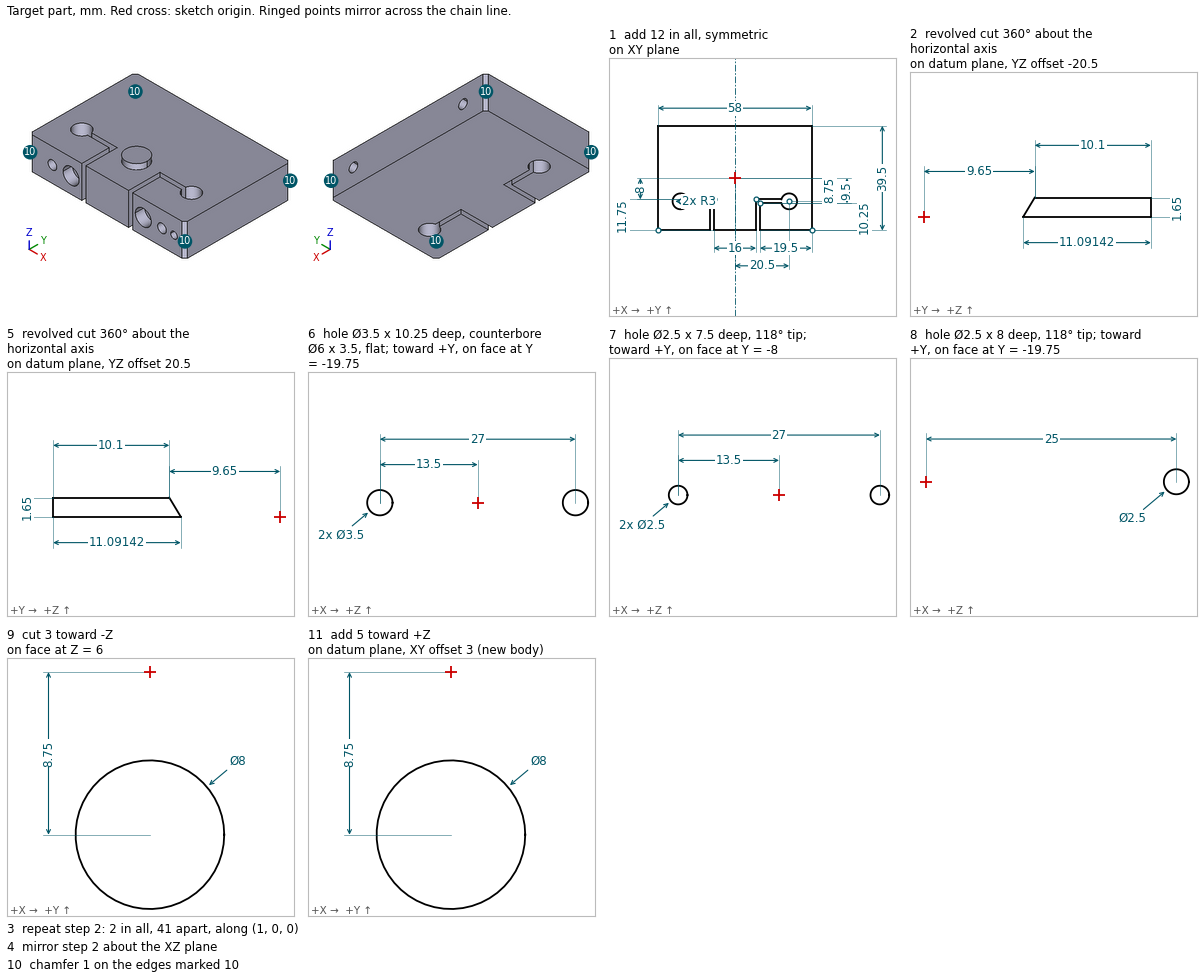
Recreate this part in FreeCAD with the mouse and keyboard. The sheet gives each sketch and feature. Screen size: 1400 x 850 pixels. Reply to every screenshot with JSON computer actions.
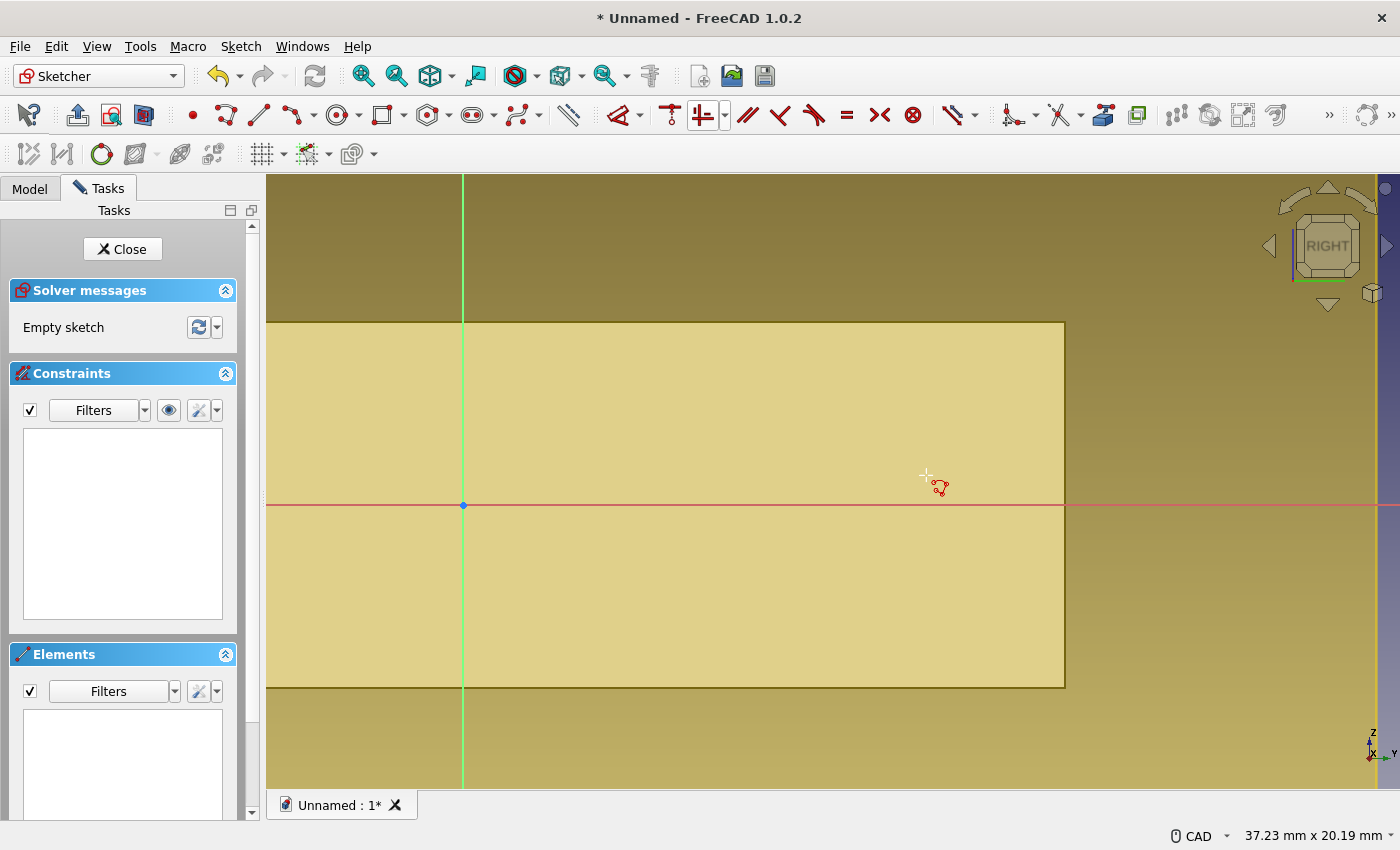
{"action": "left_click", "coordinate": [727, 505]}
{"action": "left_click", "coordinate": [1065, 496]}
{"action": "left_click", "coordinate": [1065, 455]}
{"action": "left_click", "coordinate": [757, 455]}
{"action": "left_click", "coordinate": [727, 505]}
{"action": "key", "text": "Escape"}
{"action": "key", "text": "Escape"}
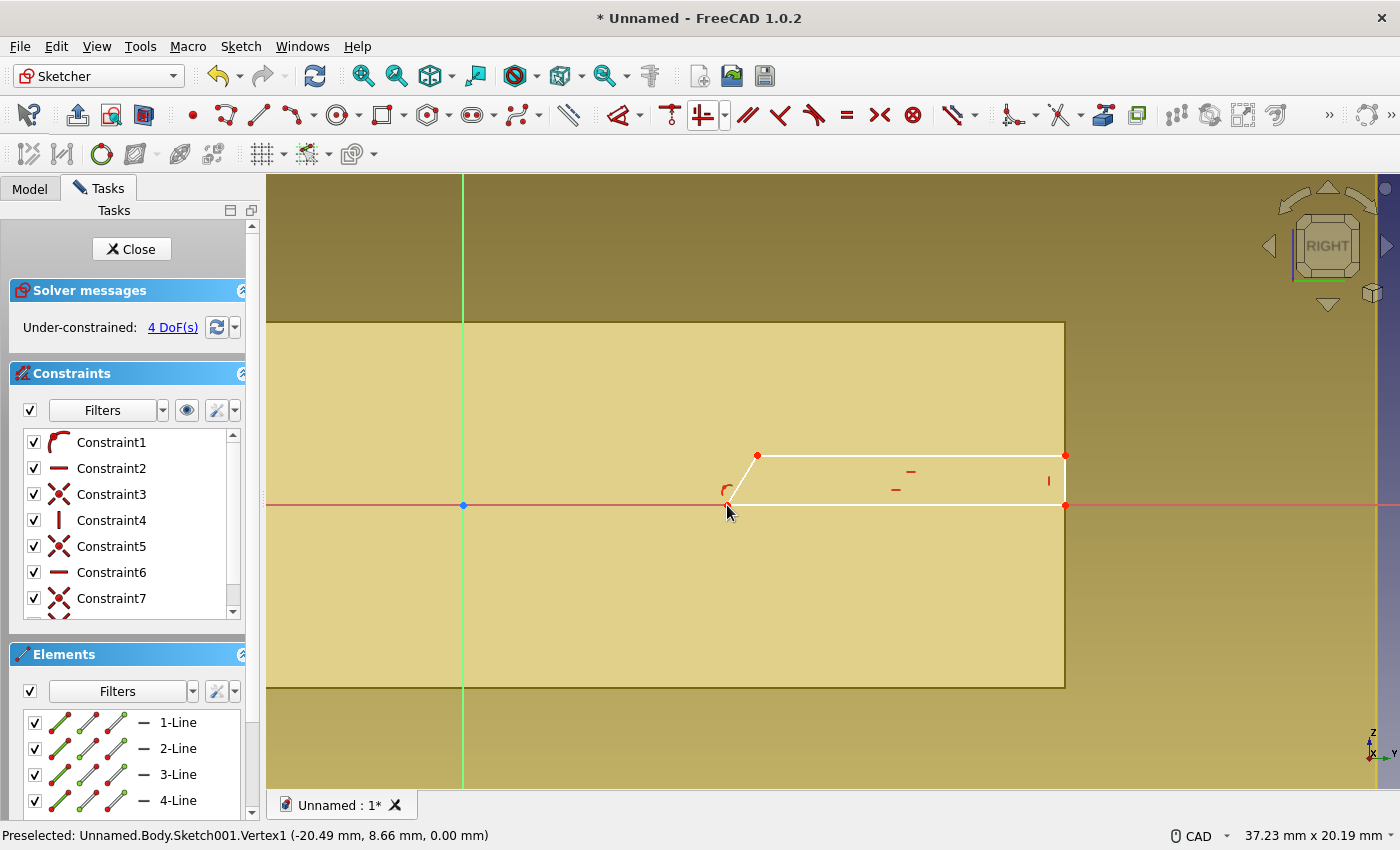
{"action": "left_click", "coordinate": [618, 116]}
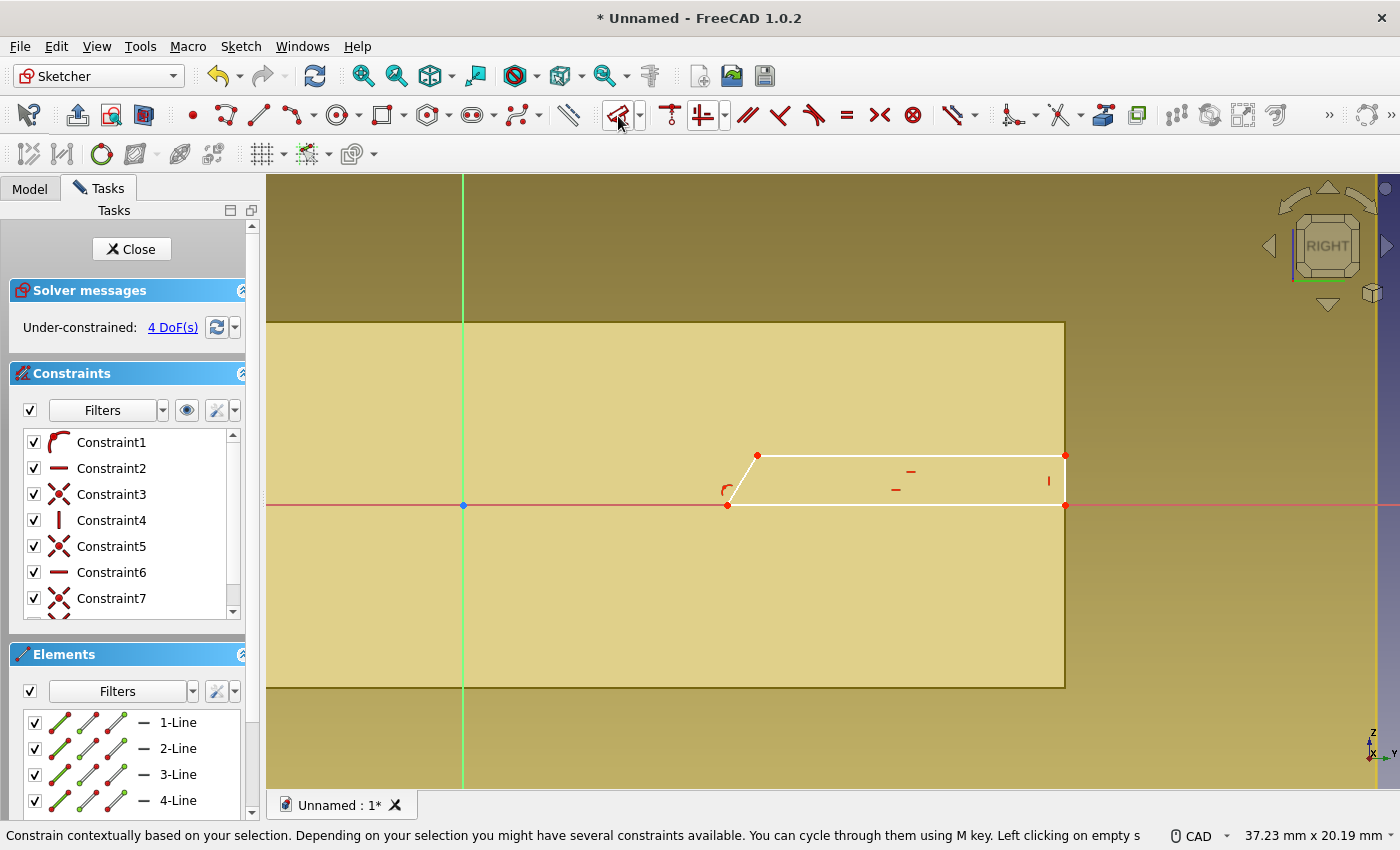
{"action": "left_click", "coordinate": [1065, 490]}
{"action": "left_click", "coordinate": [1099, 481]}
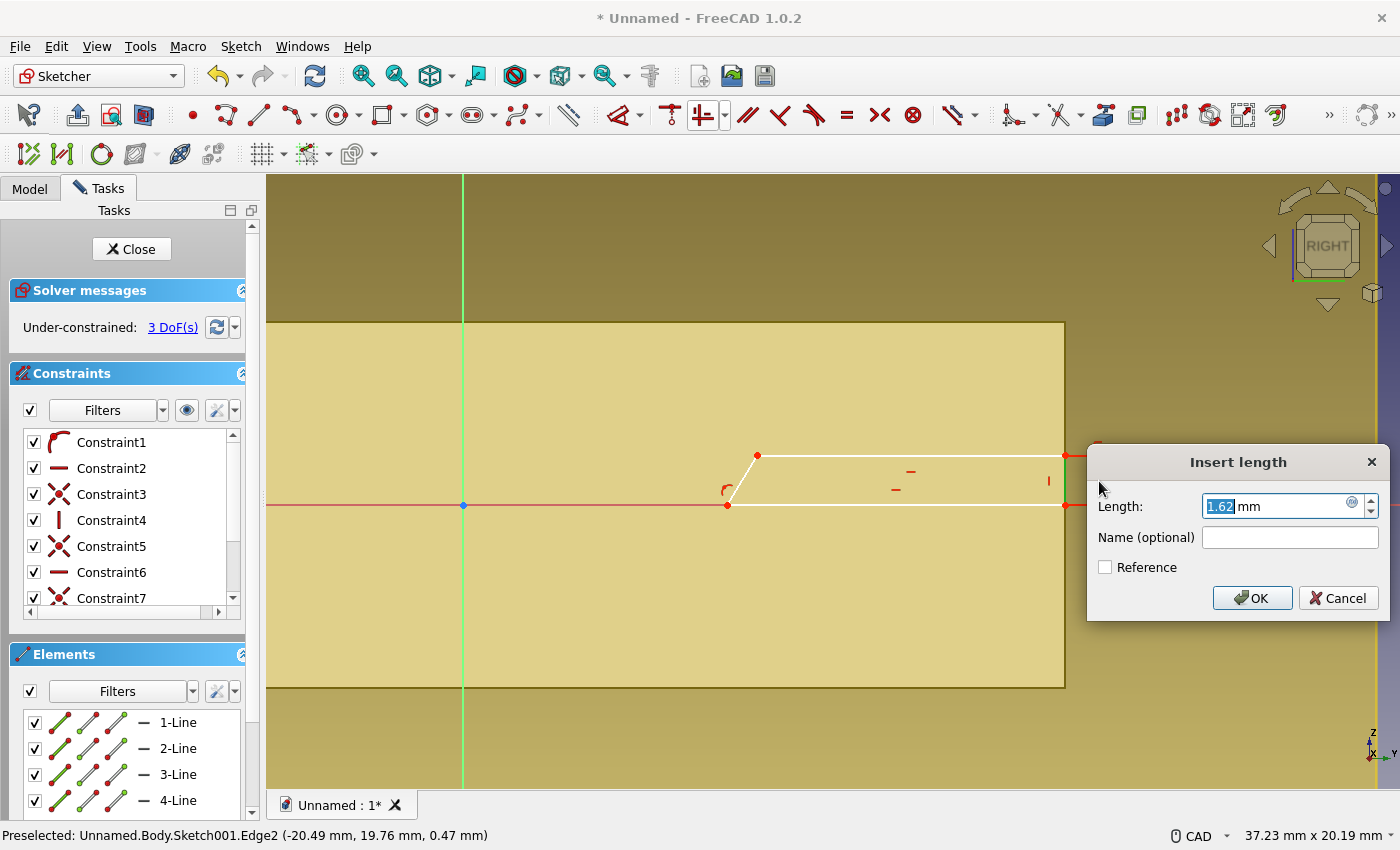
{"action": "type", "text": "1.65"}
{"action": "key", "text": "Return"}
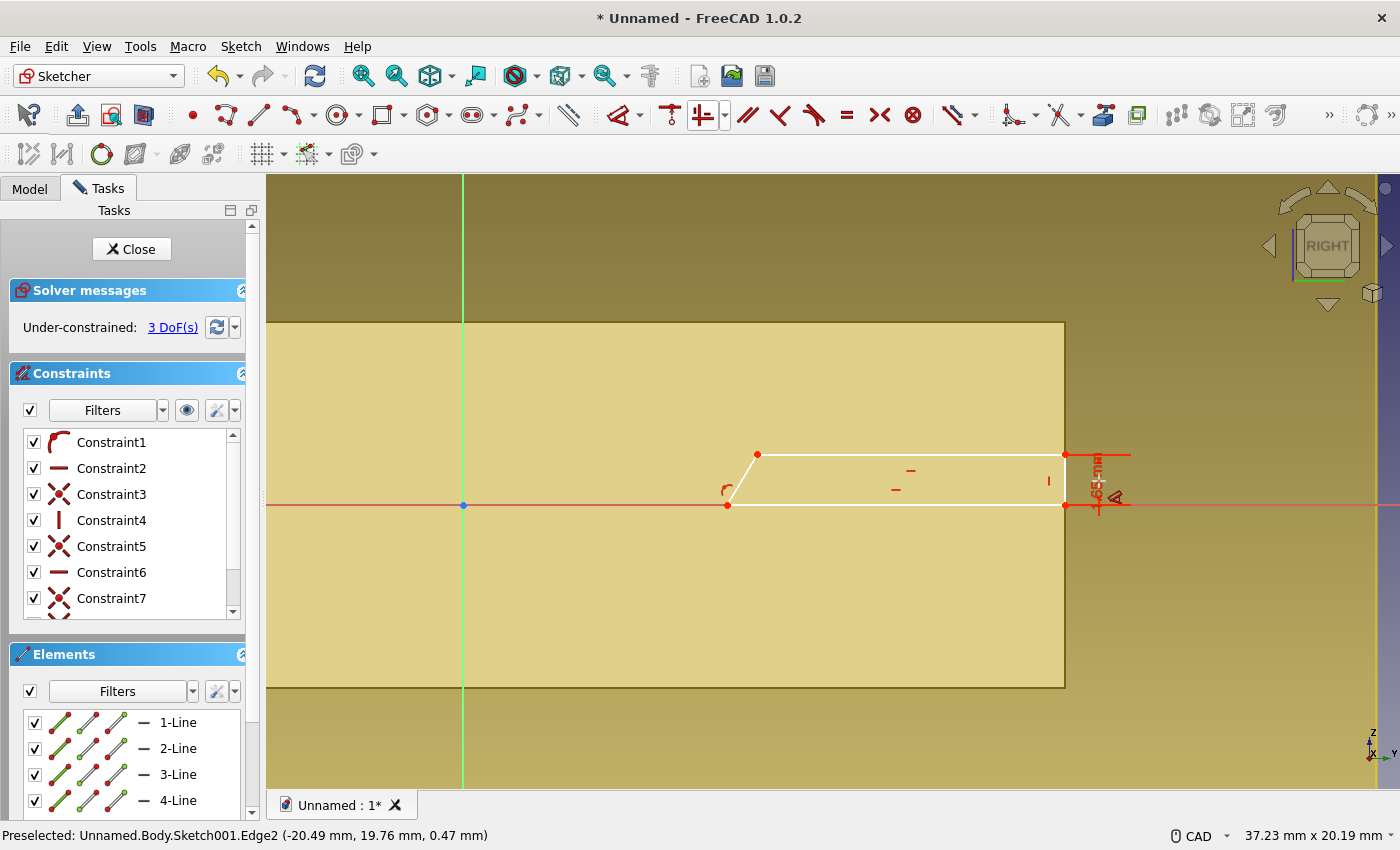
{"action": "left_click", "coordinate": [973, 455]}
{"action": "left_click", "coordinate": [911, 421]}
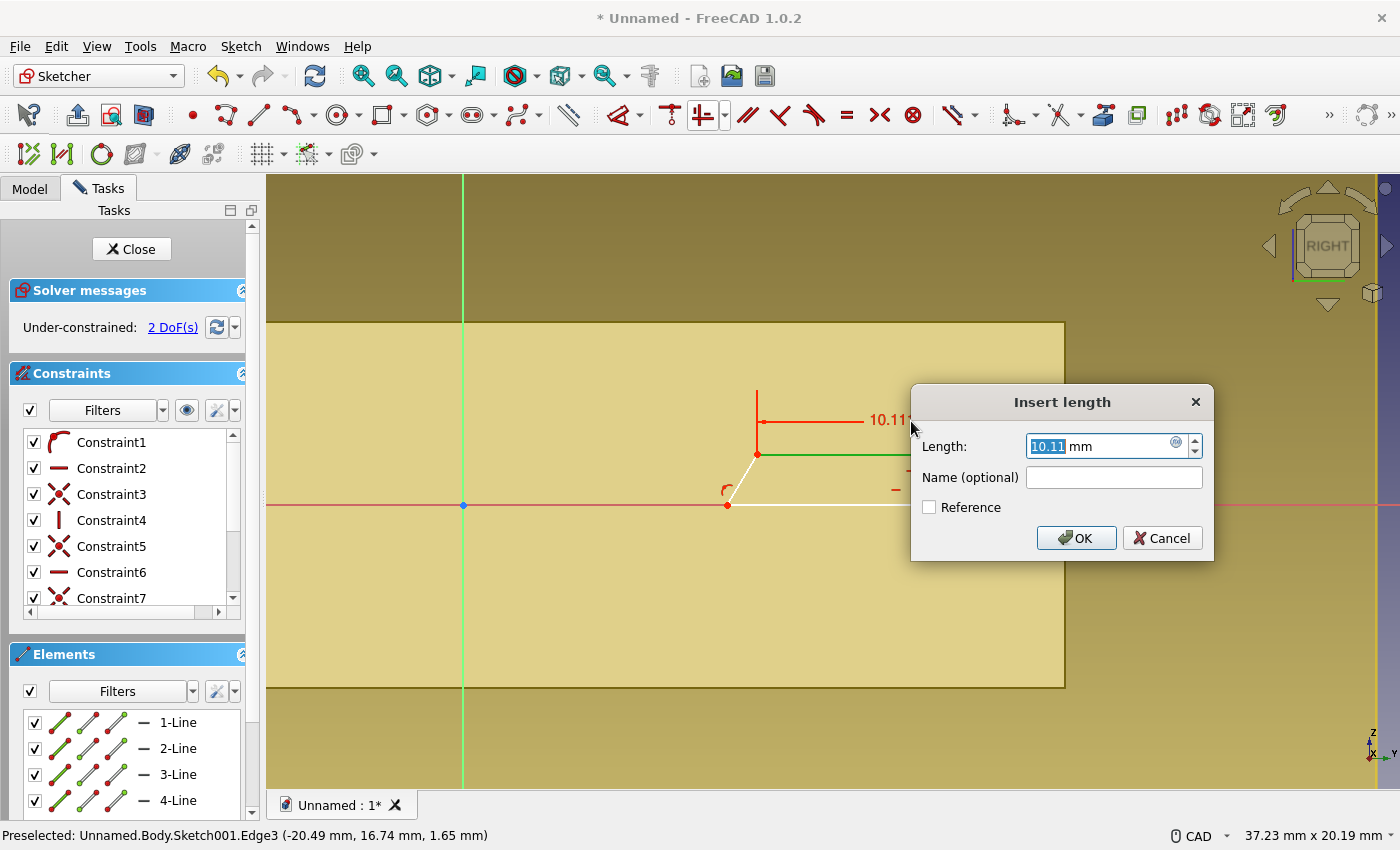
{"action": "type", "text": "10.1"}
{"action": "key", "text": "Return"}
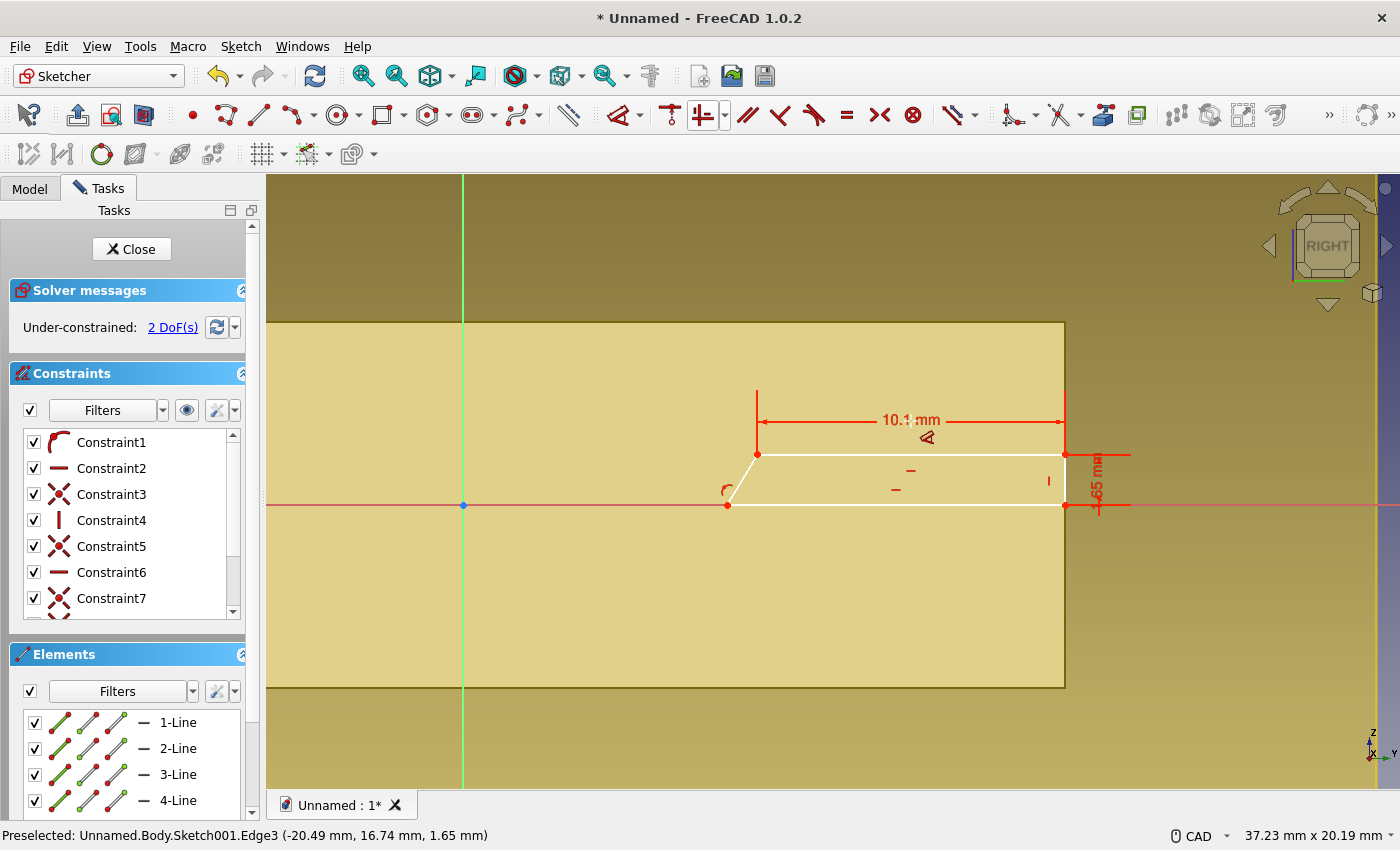
{"action": "left_click", "coordinate": [757, 455]}
{"action": "left_click", "coordinate": [610, 539]}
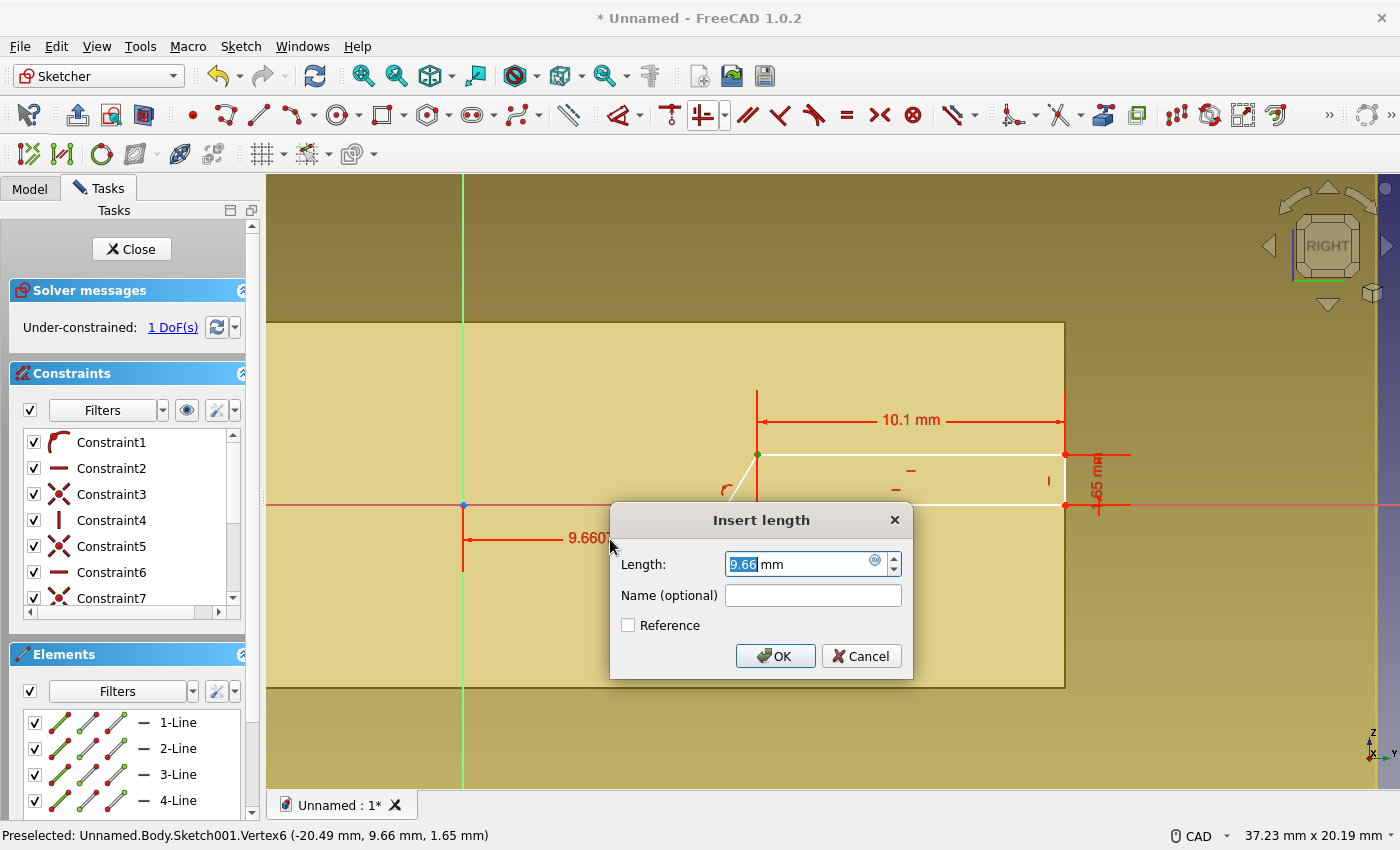
{"action": "type", "text": "9.65"}
{"action": "key", "text": "Return"}